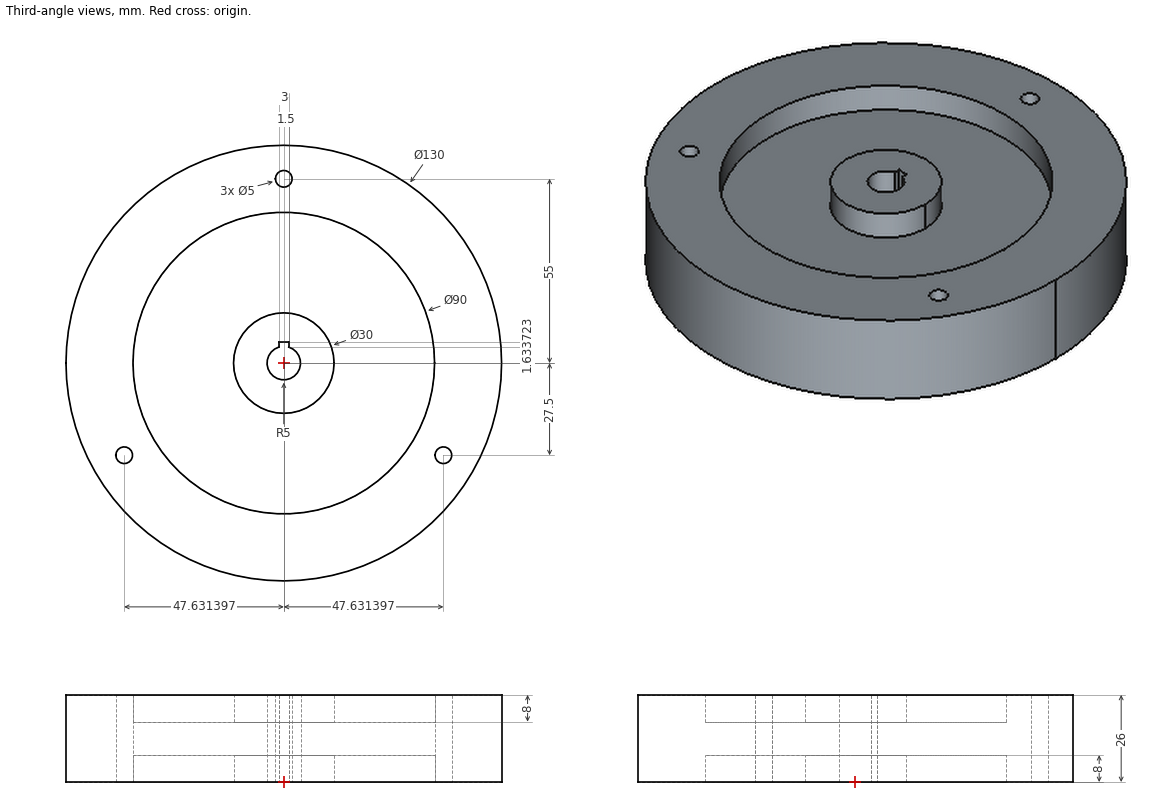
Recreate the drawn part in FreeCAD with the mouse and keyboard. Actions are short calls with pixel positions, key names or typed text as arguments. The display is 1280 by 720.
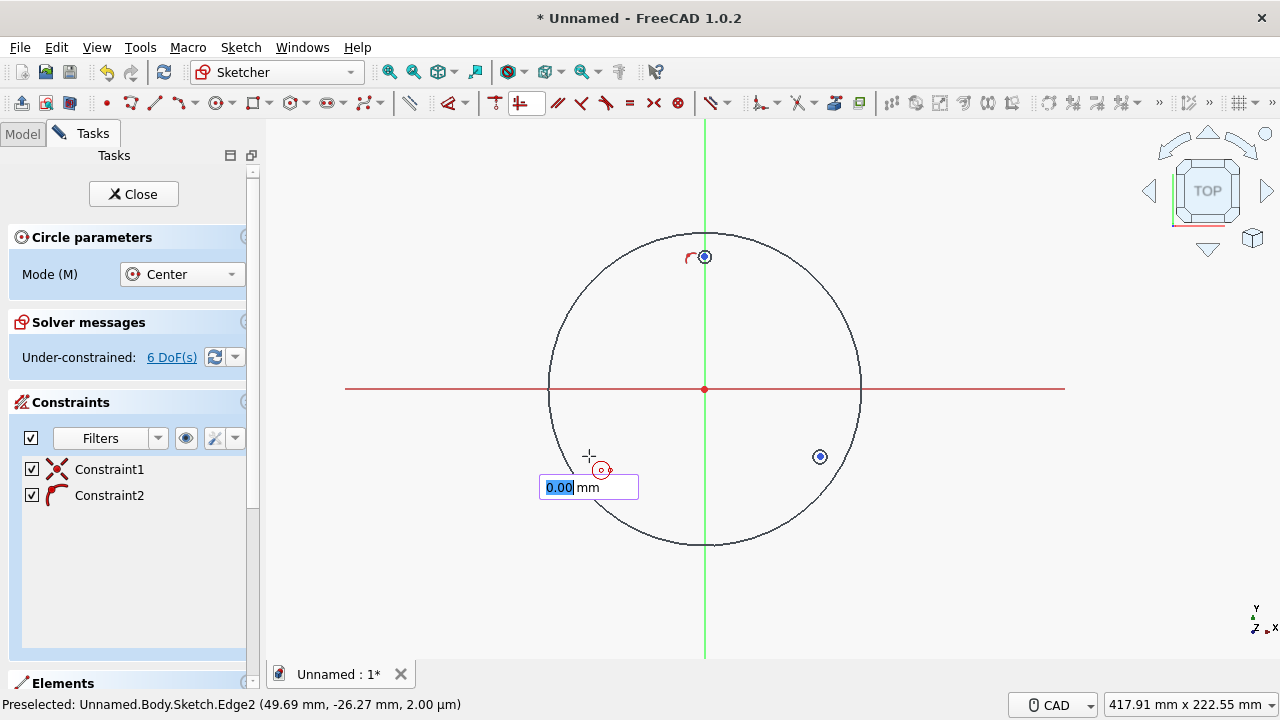
scroll(594, 452, up, 5)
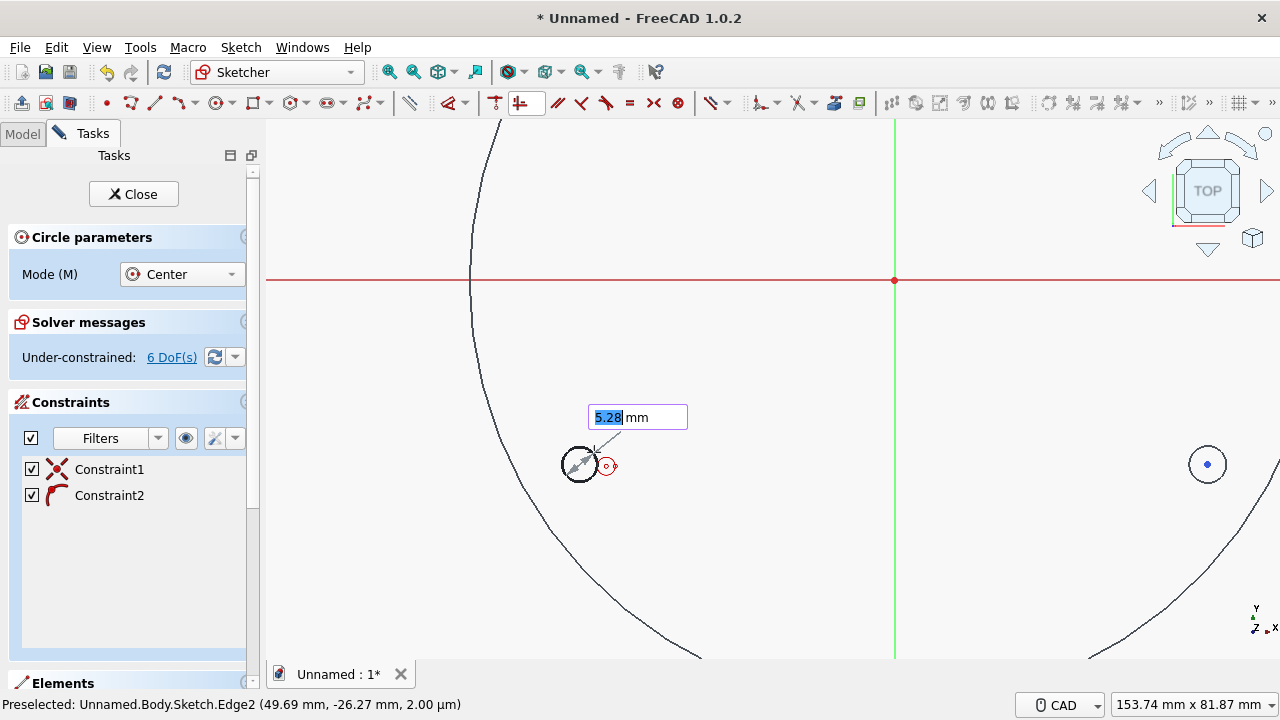
click(592, 450)
key(Escape)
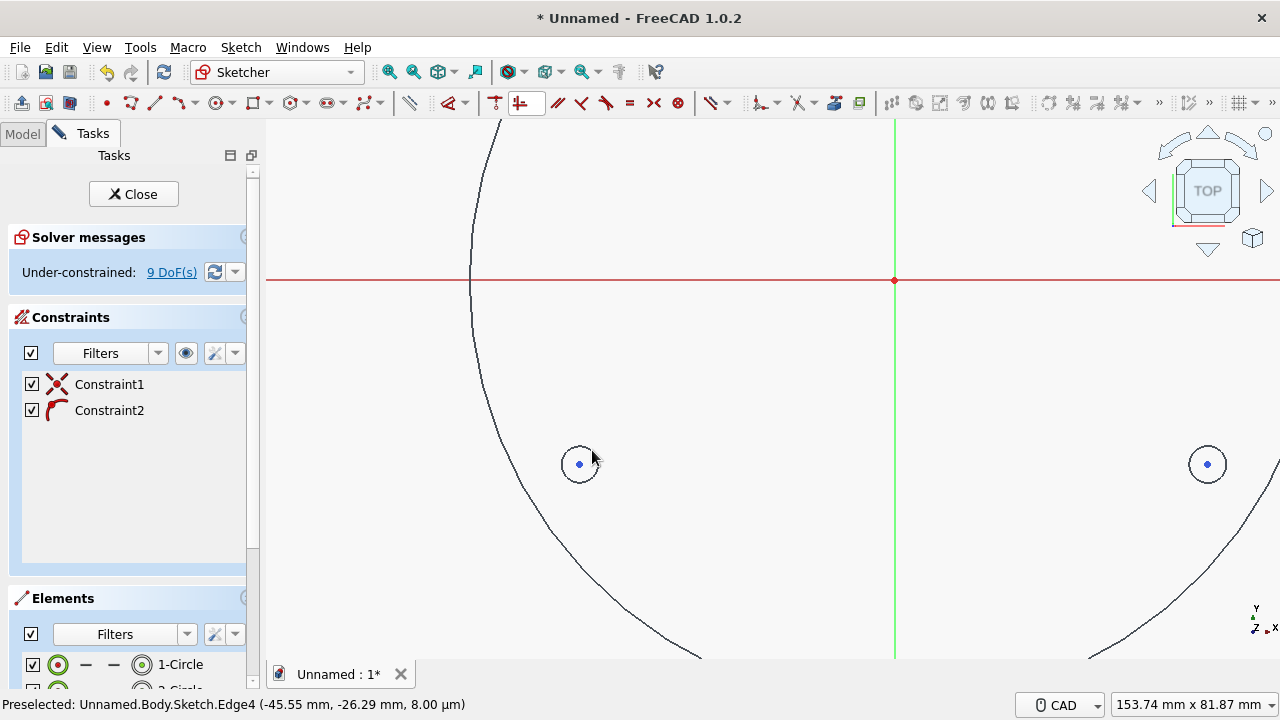
scroll(594, 452, down, 5)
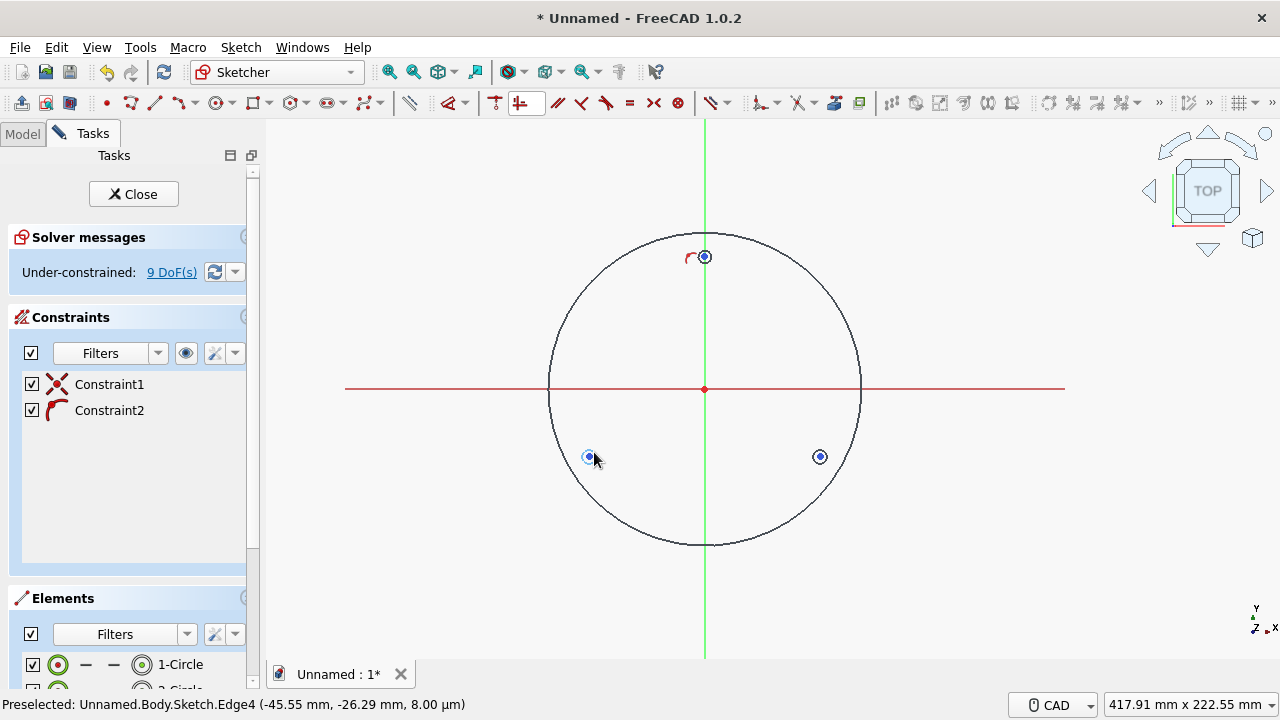
scroll(709, 252, up, 6)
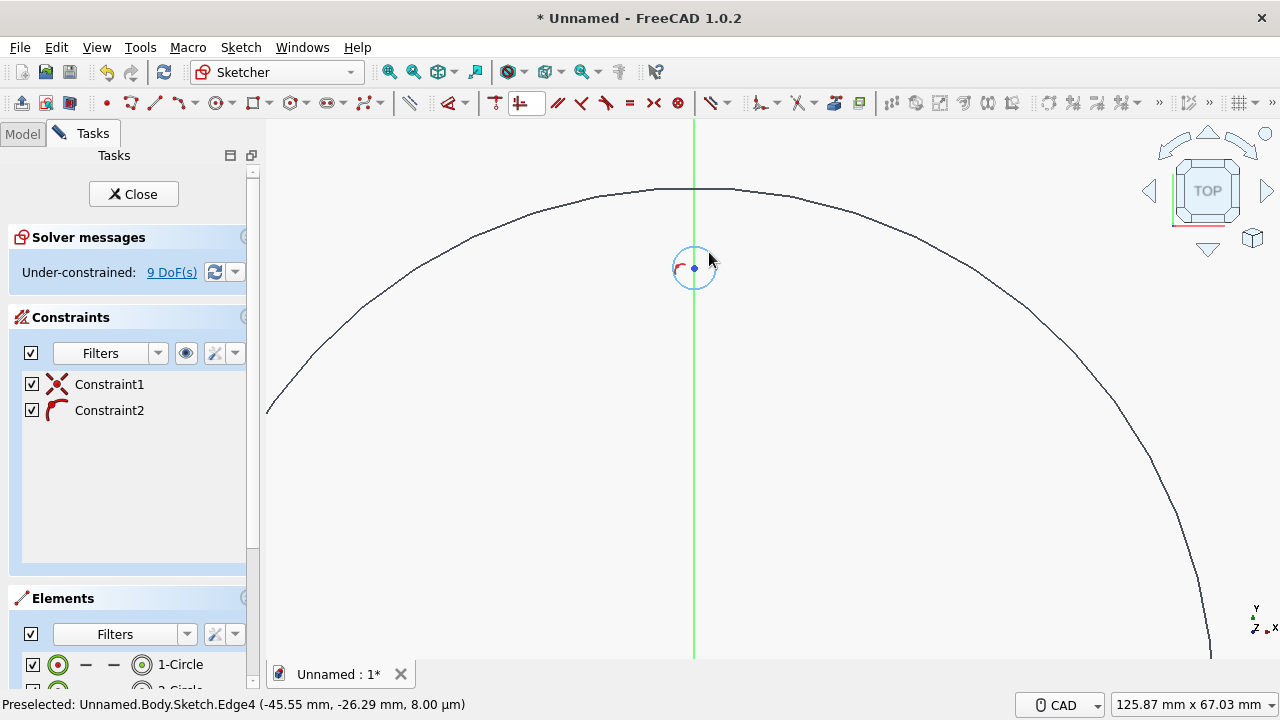
click(710, 253)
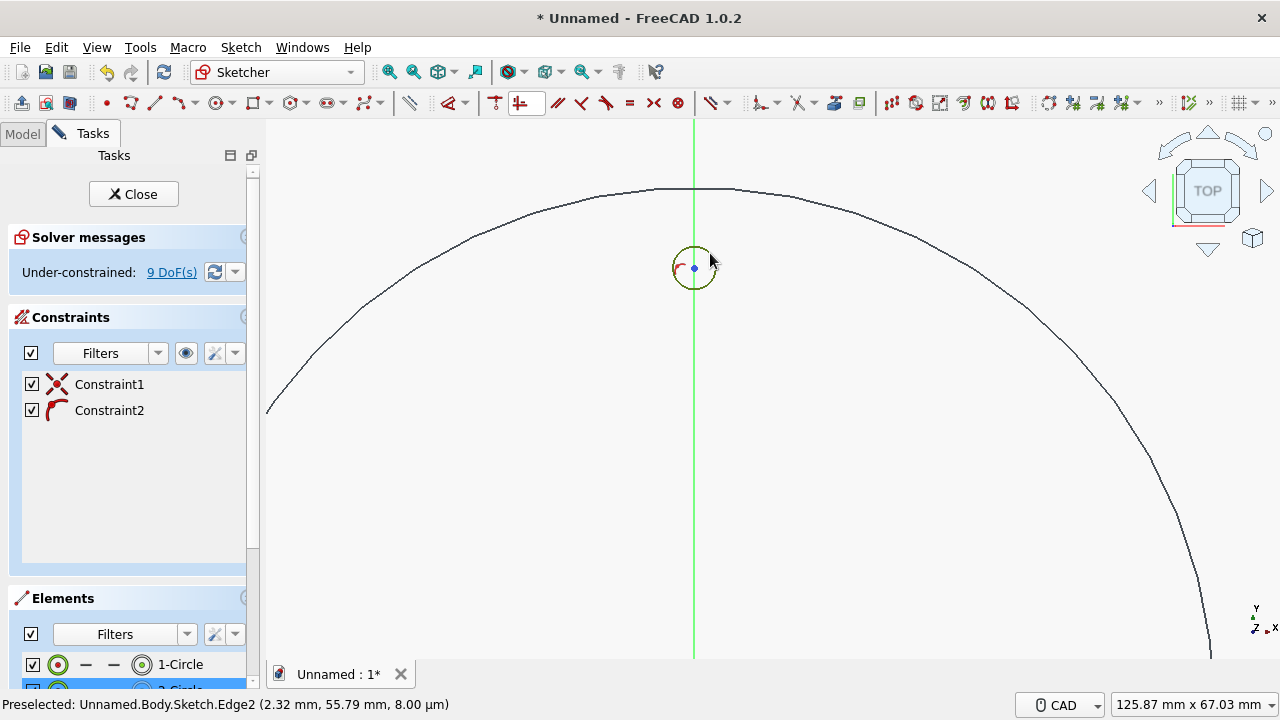
scroll(709, 252, down, 6)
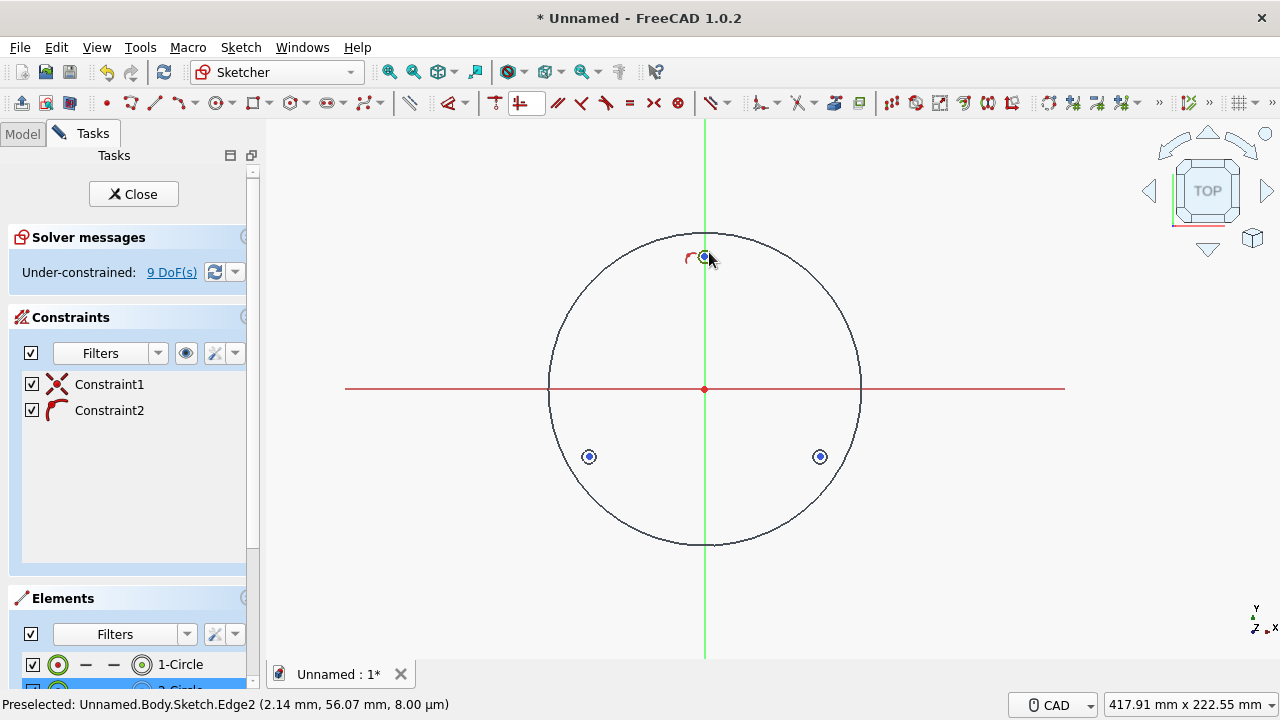
scroll(825, 452, up, 4)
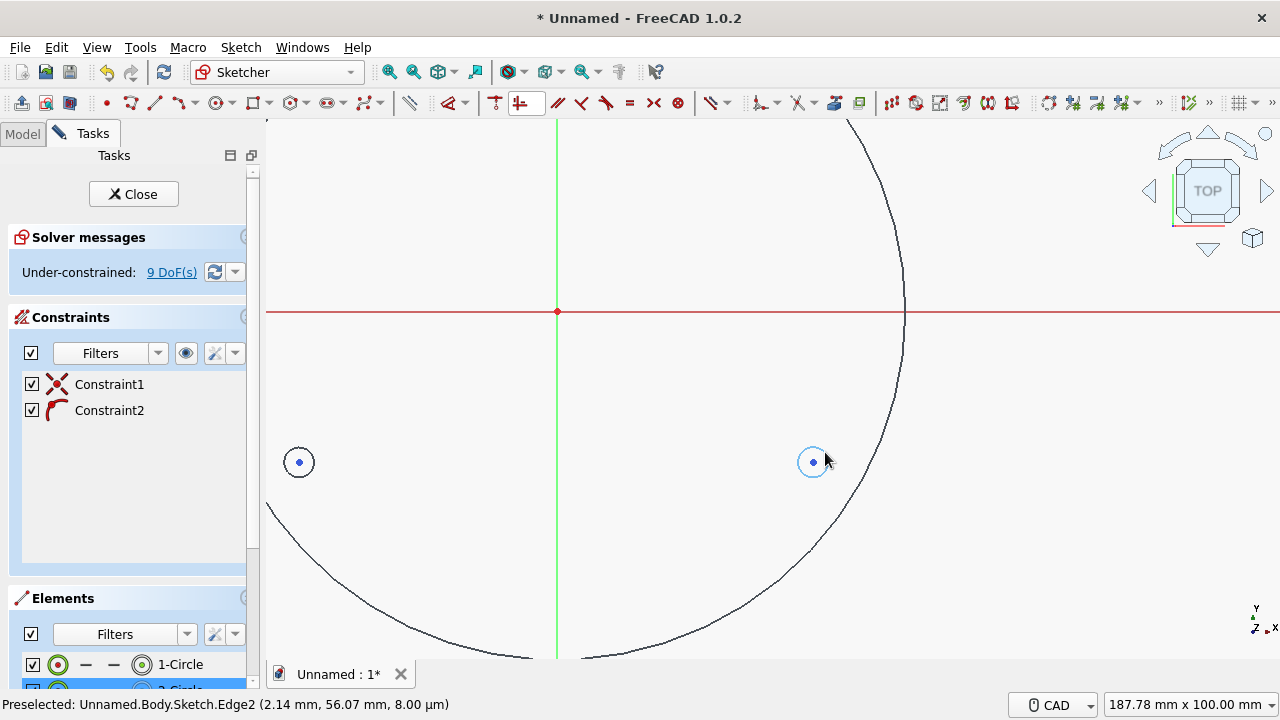
click(824, 452)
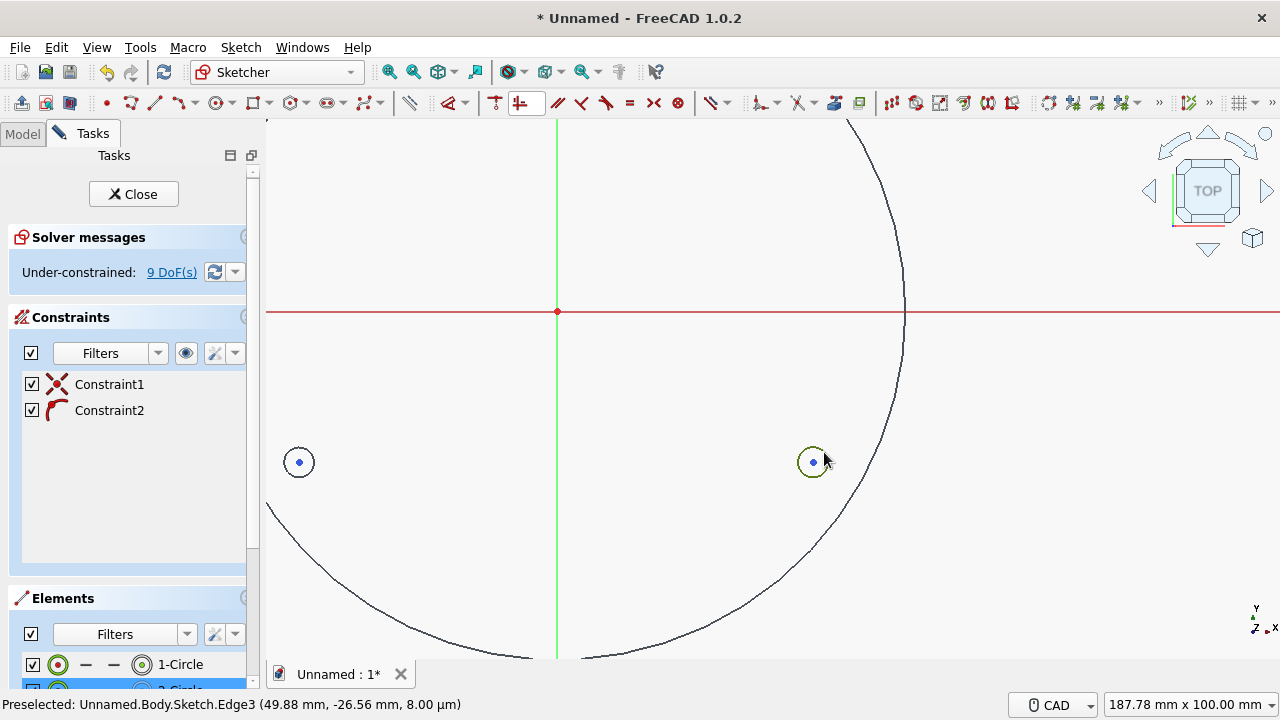
click(310, 452)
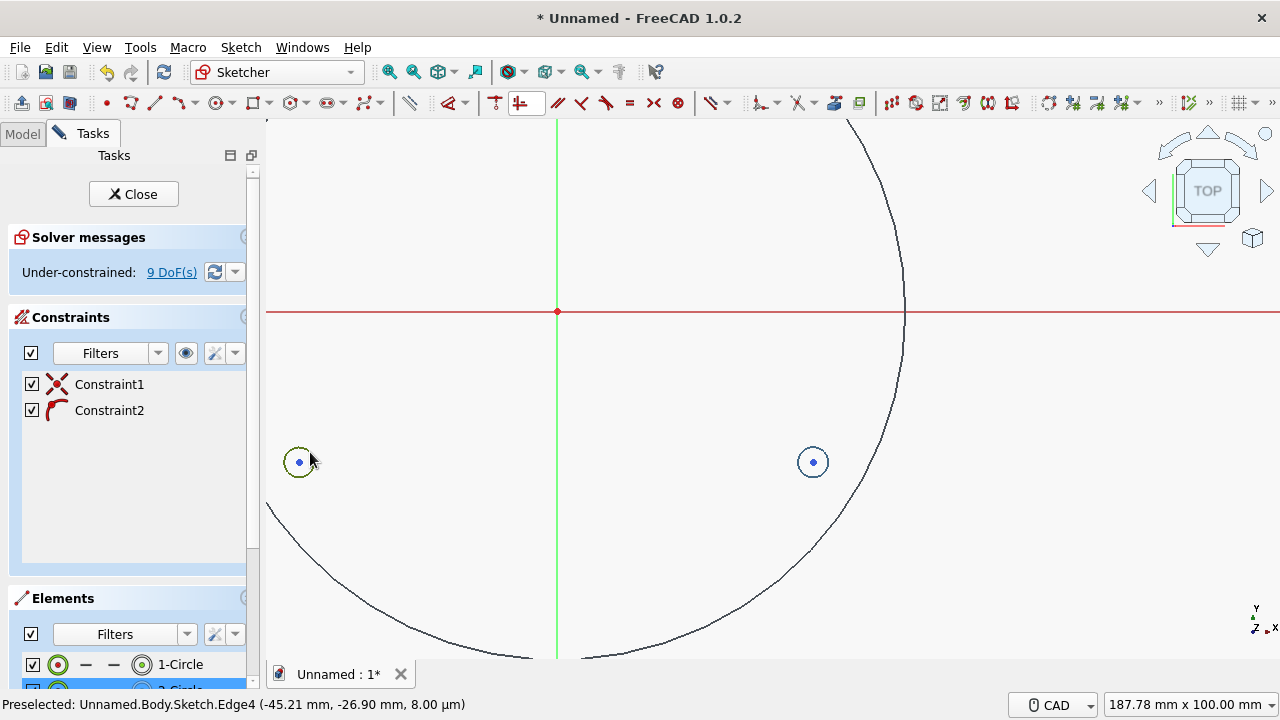
key(e)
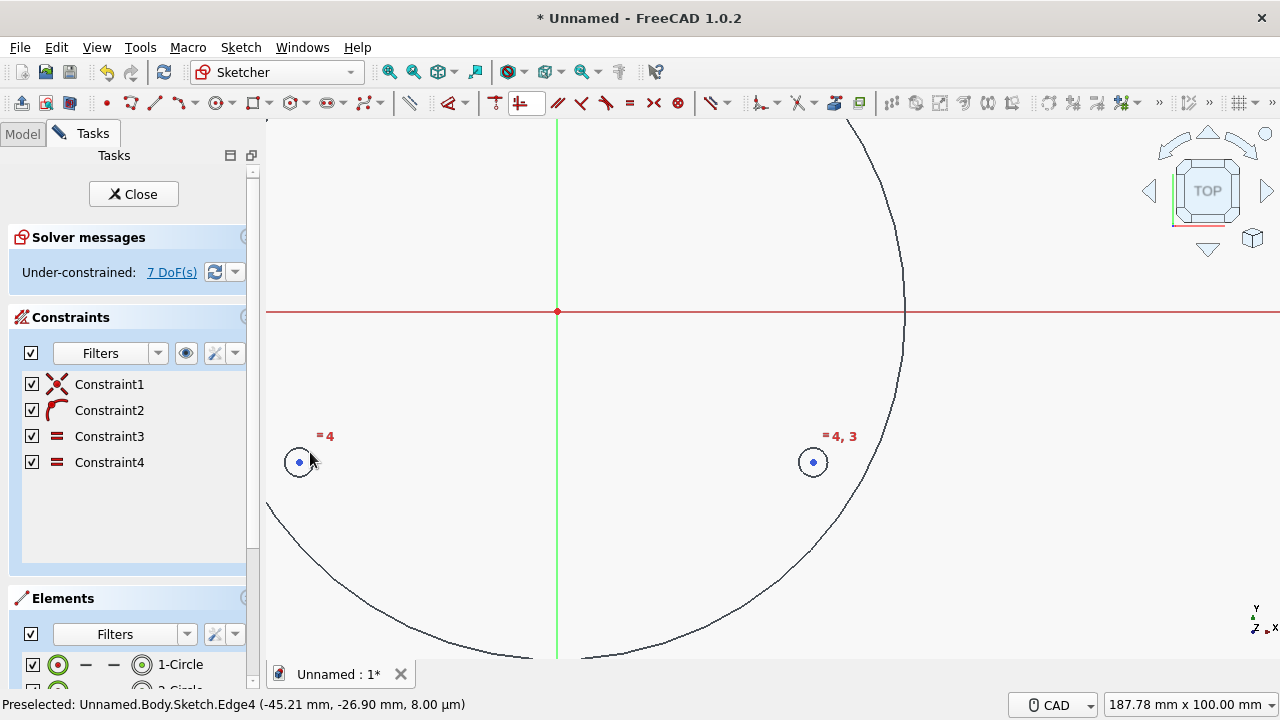
click(813, 462)